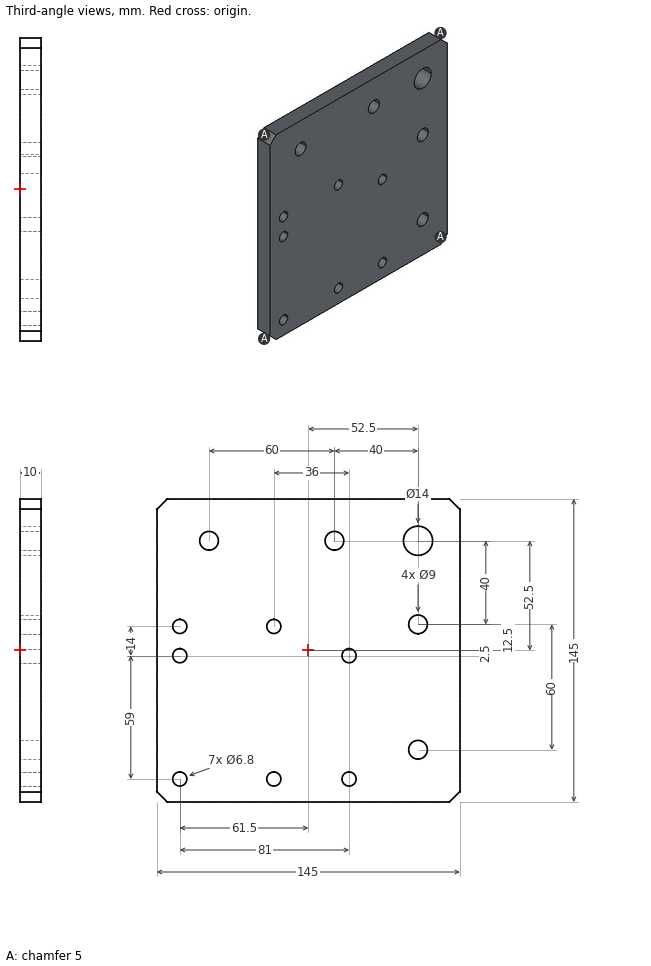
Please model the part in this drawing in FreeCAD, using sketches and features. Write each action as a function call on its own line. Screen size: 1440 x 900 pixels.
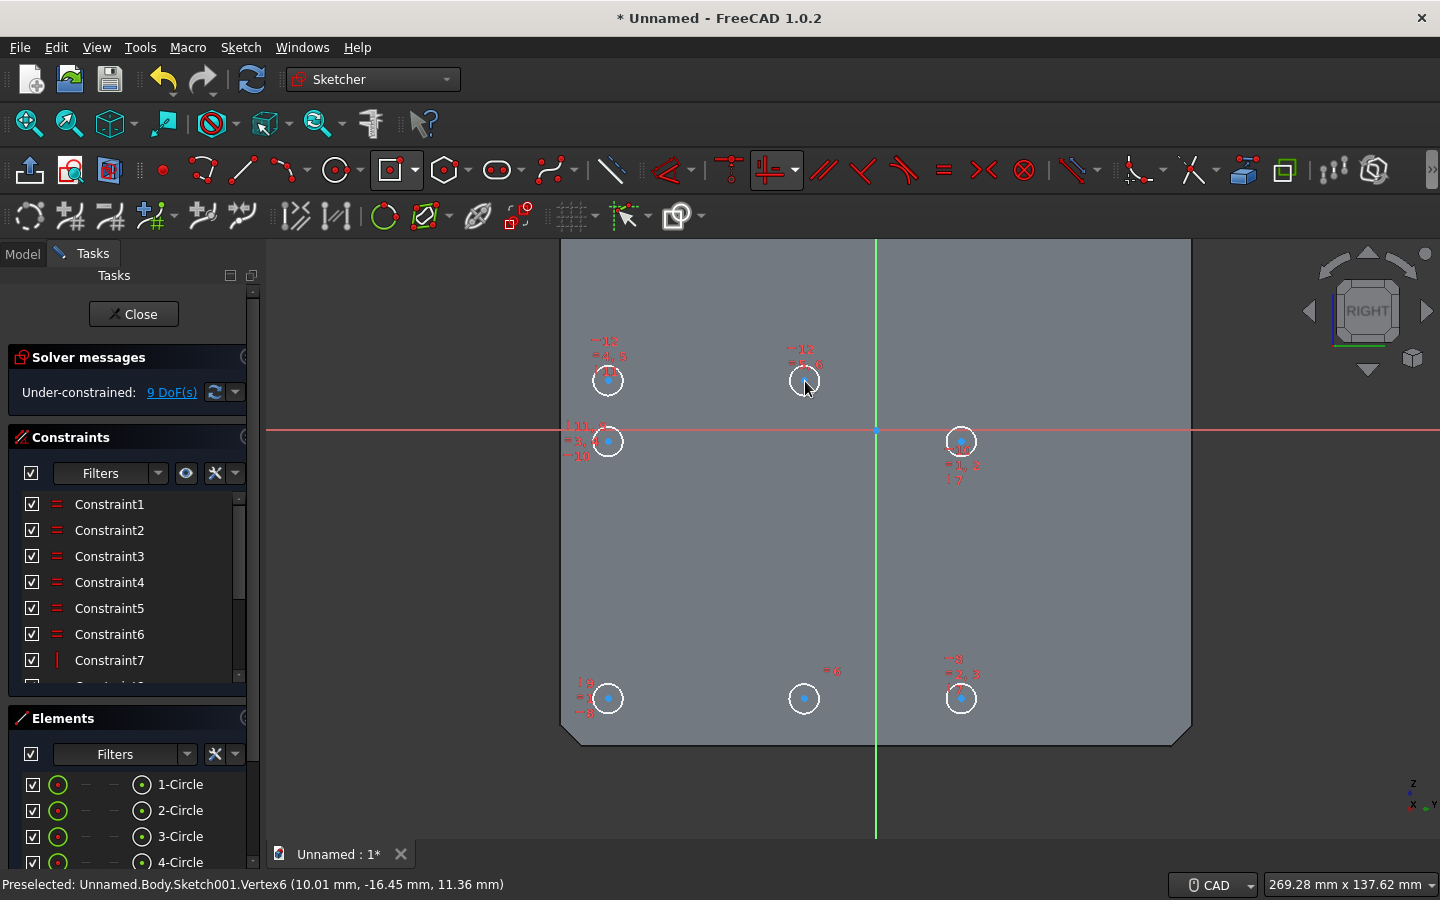
click(805, 381)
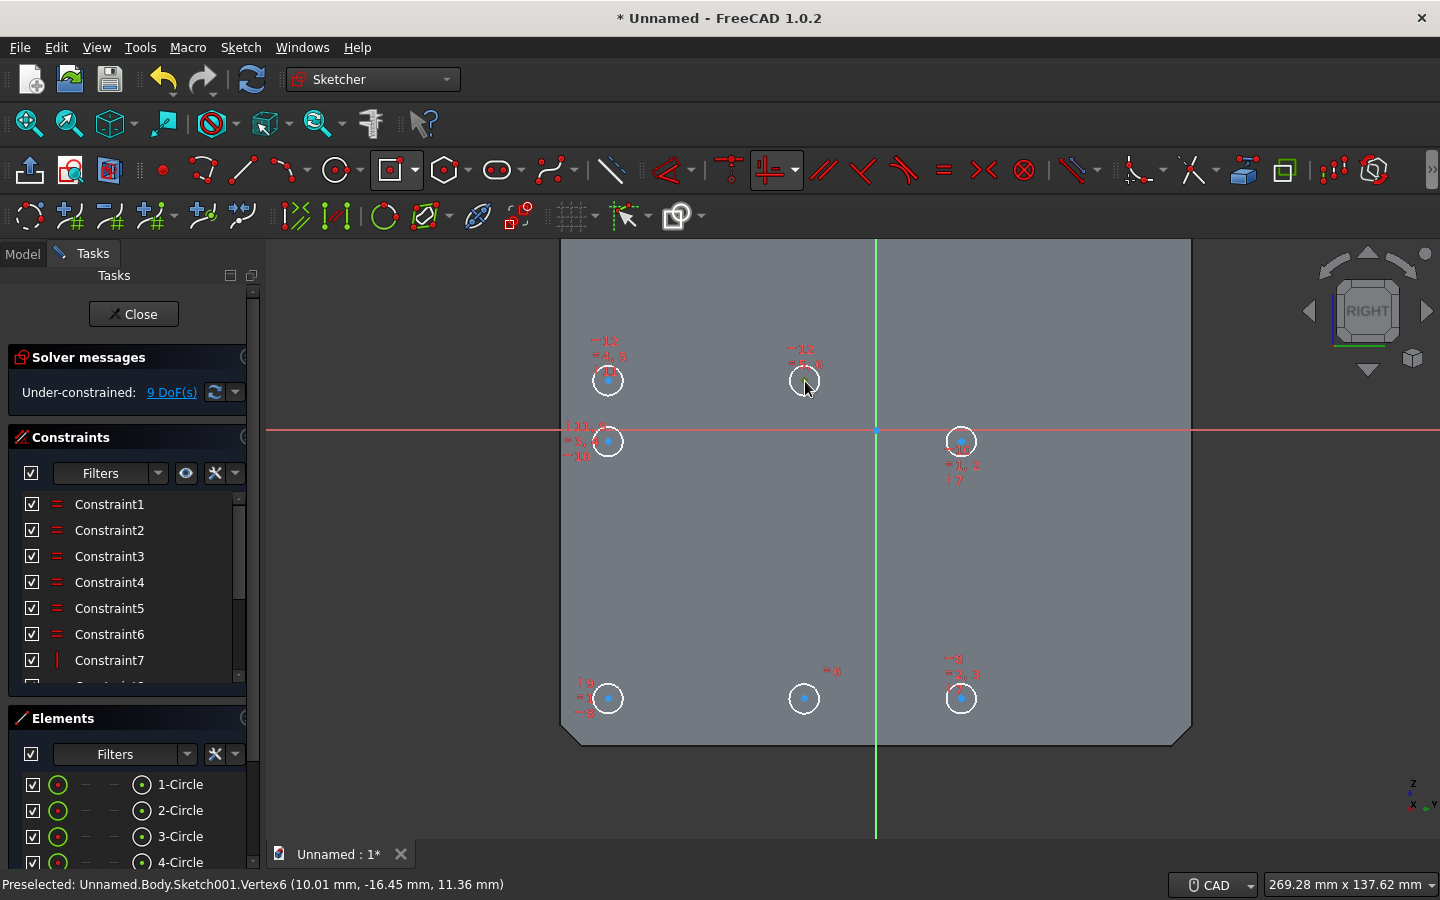
click(804, 699)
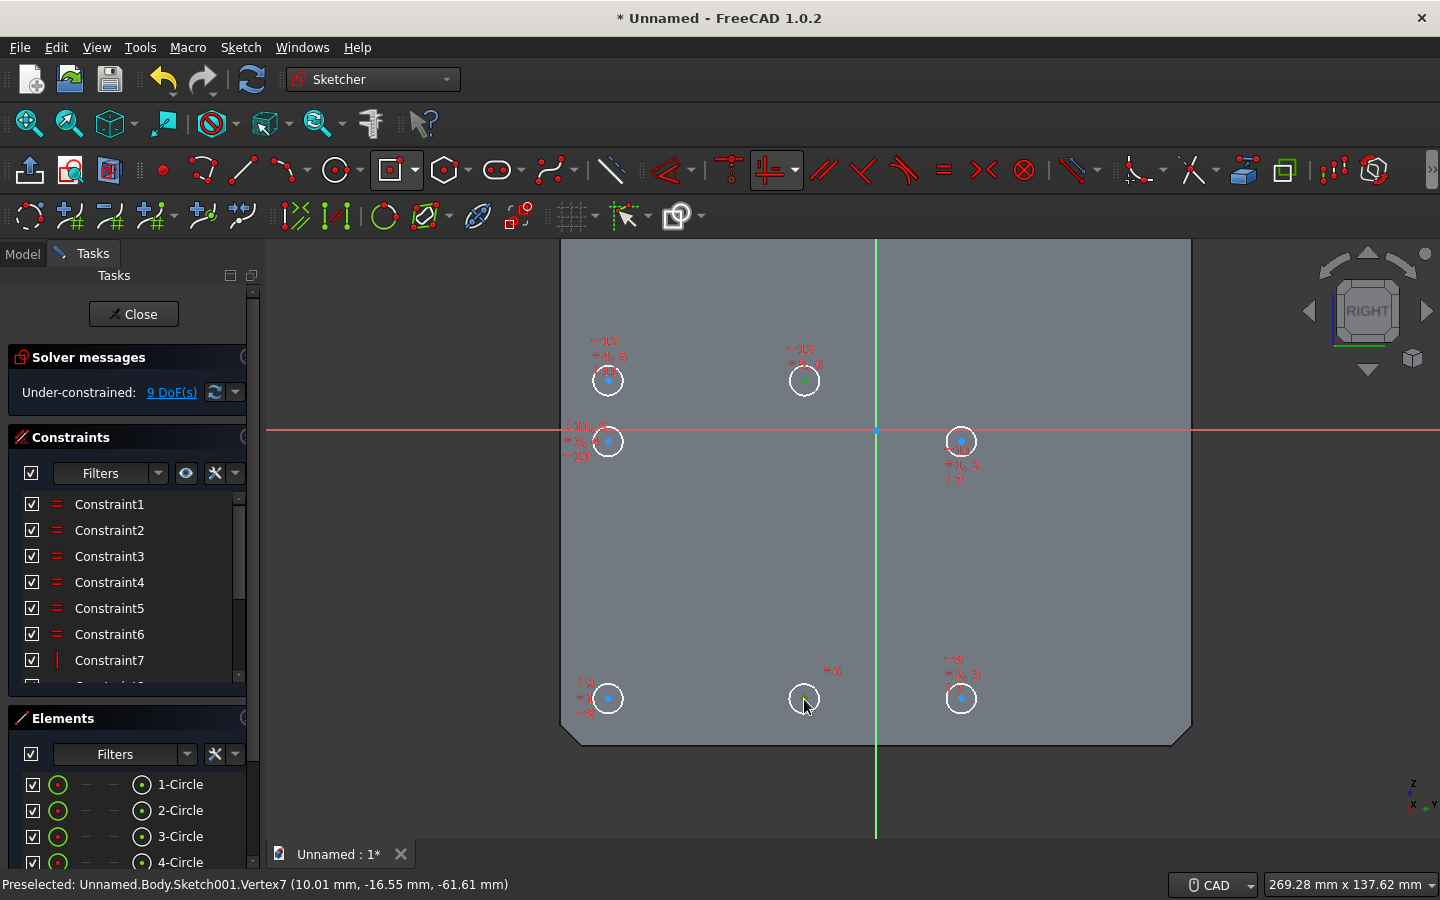
key(v)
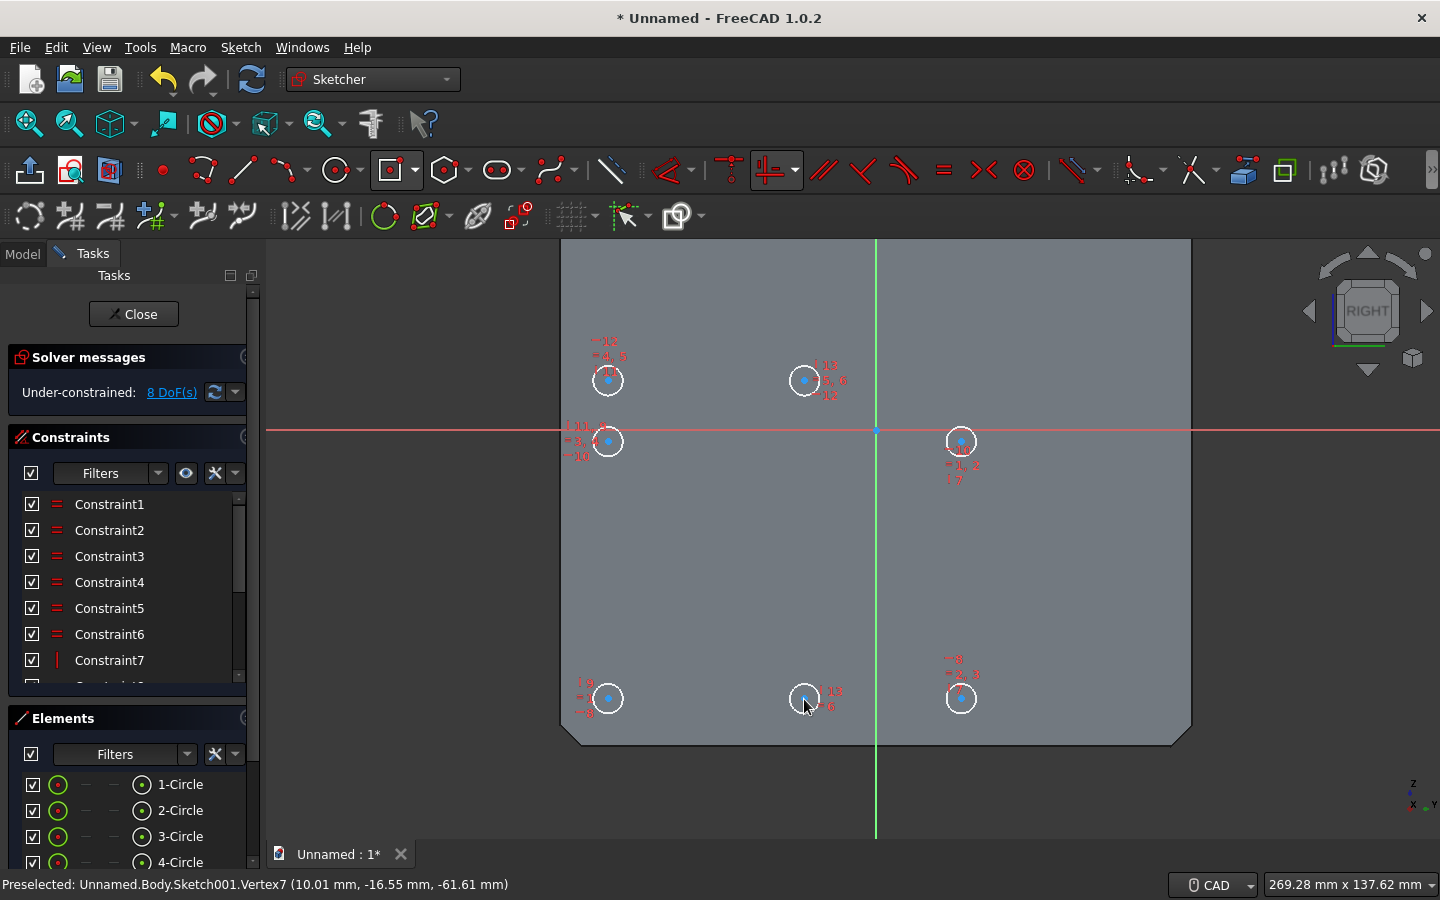
click(961, 699)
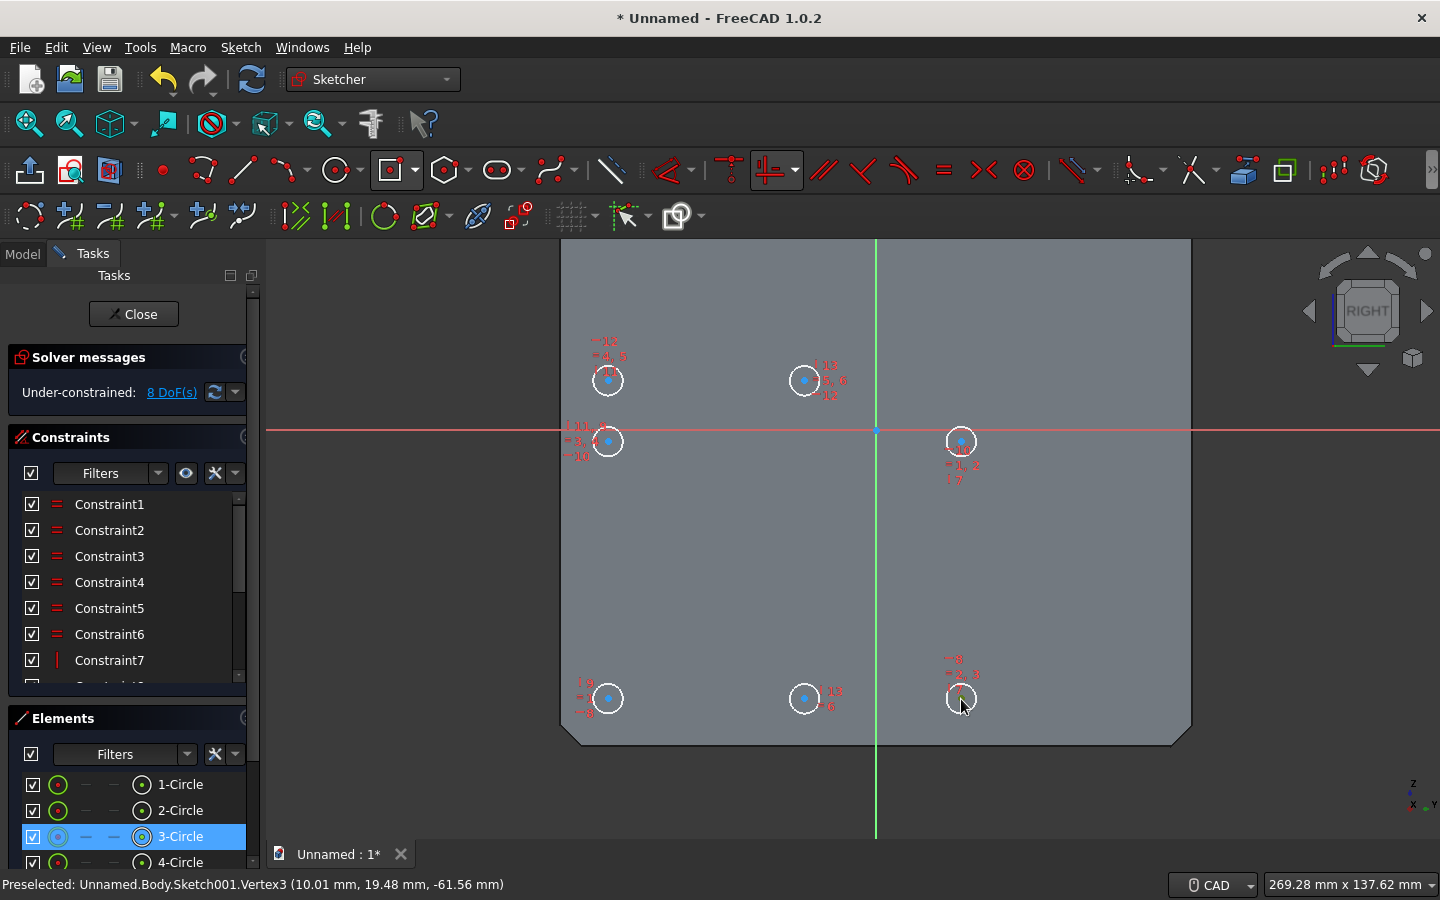
click(805, 699)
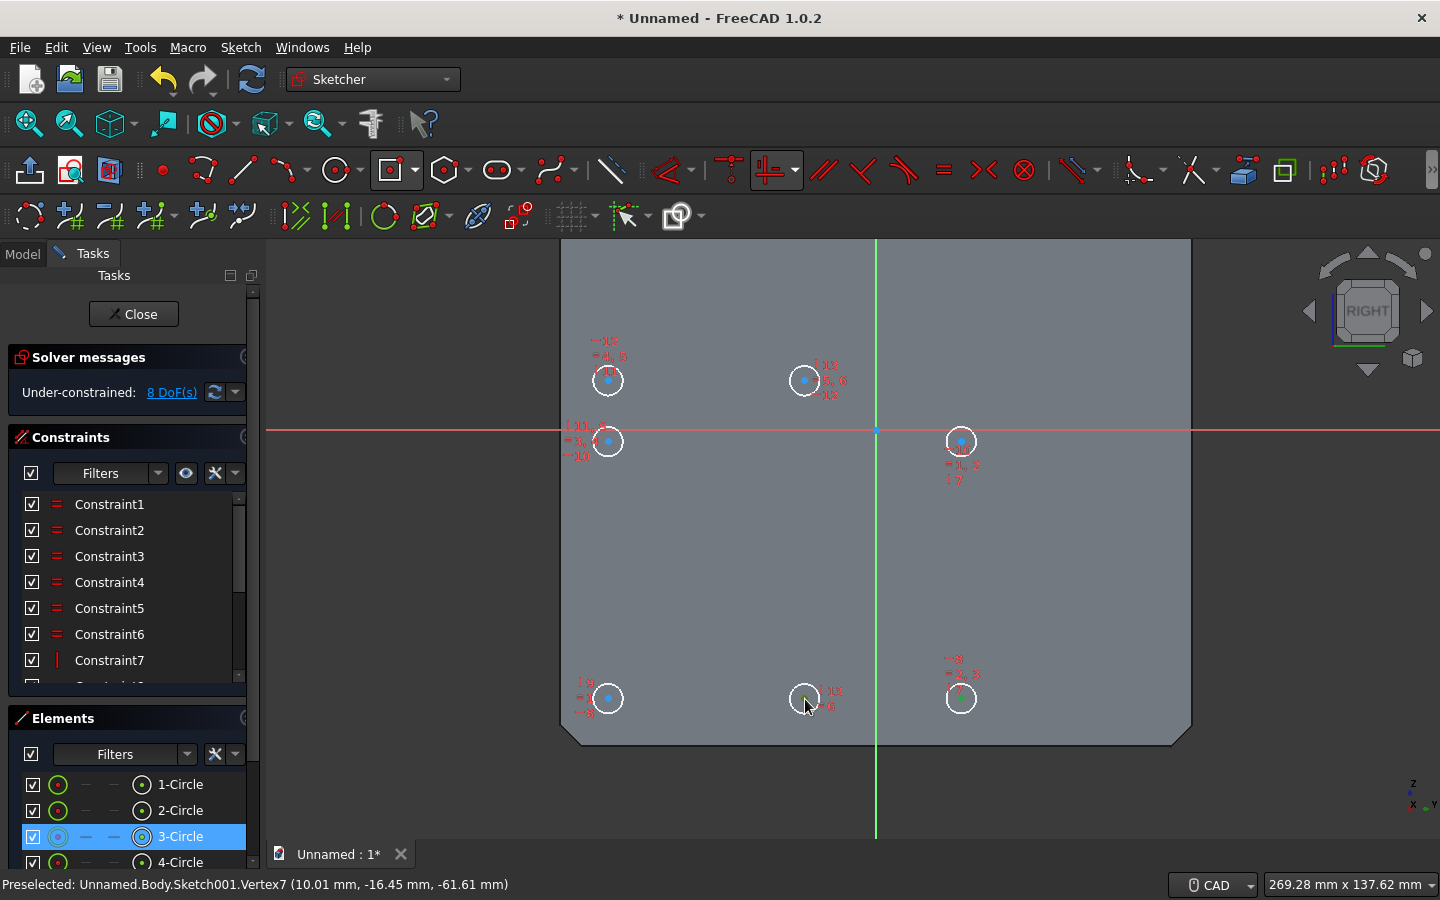
click(798, 170)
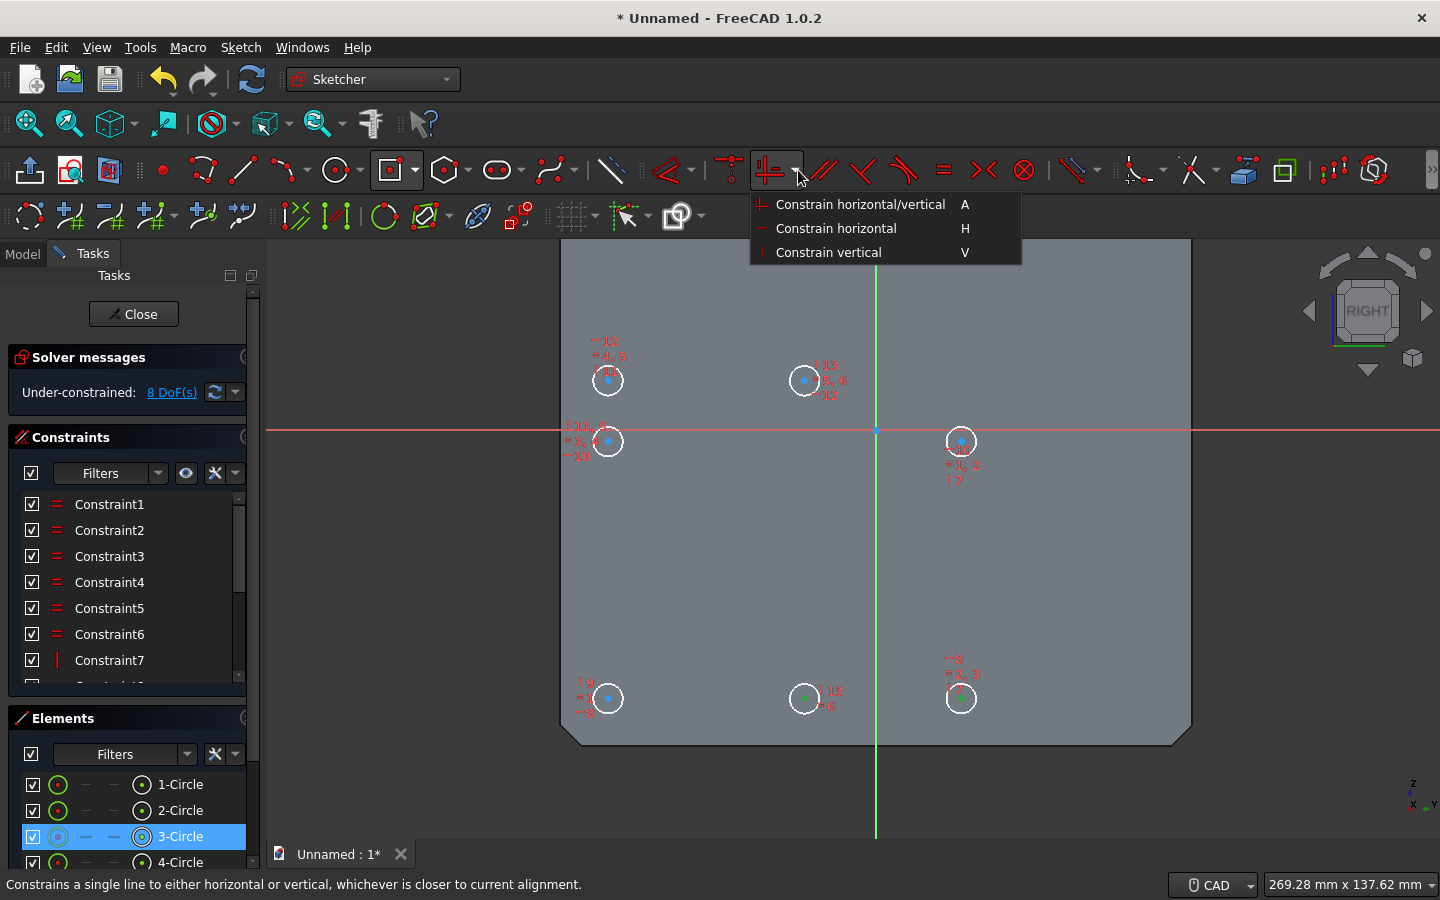
click(886, 228)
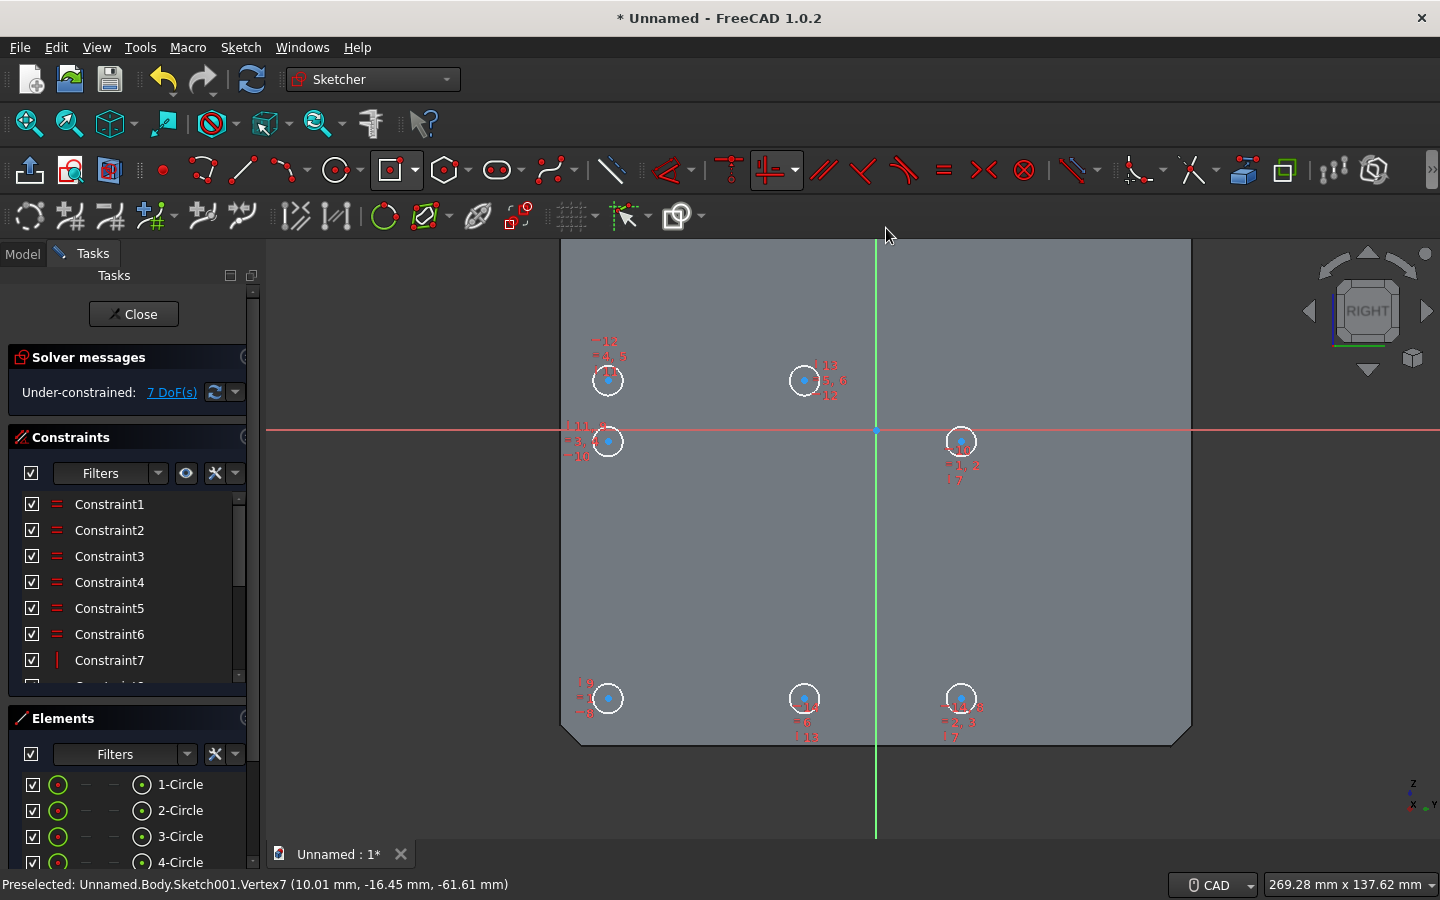
key(d)